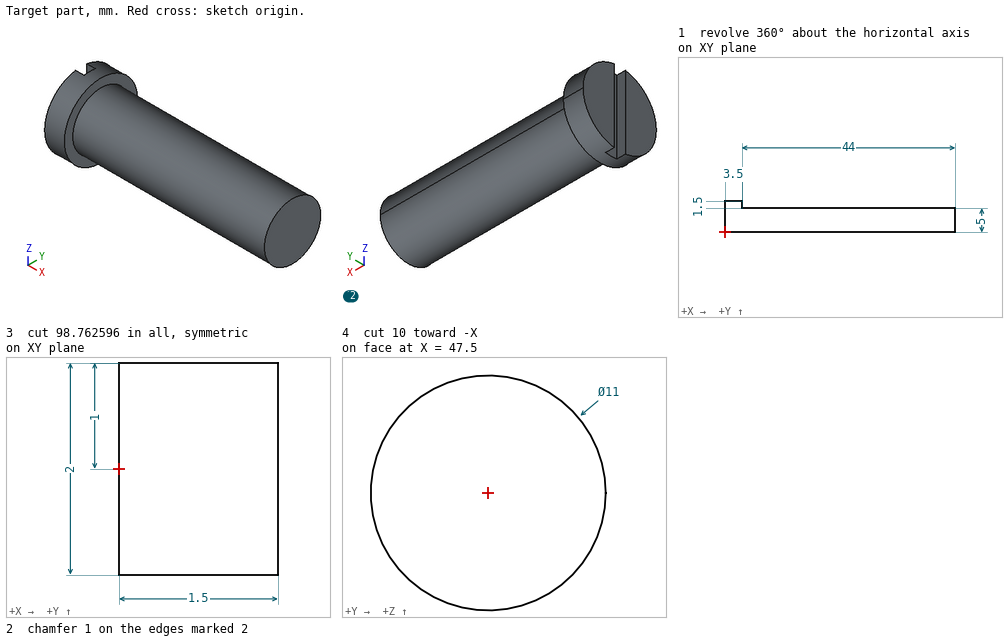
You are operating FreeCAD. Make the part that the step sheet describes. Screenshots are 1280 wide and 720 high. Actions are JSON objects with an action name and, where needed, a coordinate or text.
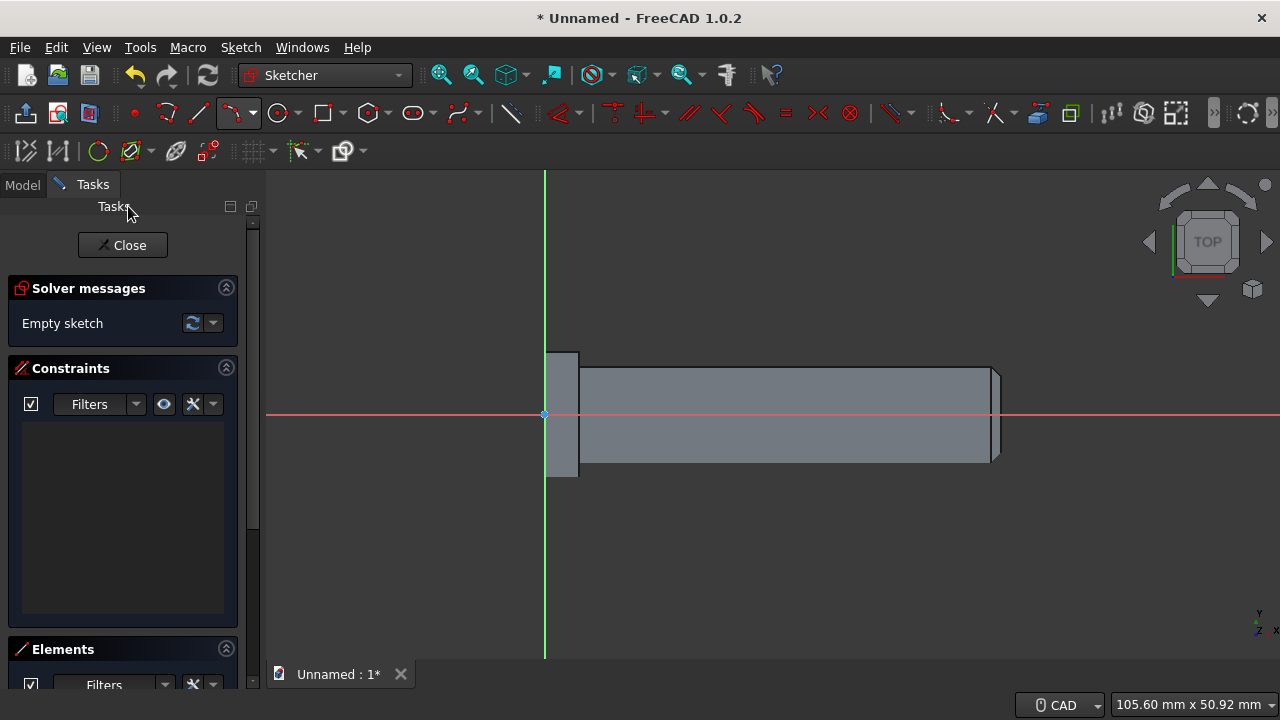
{"action": "scroll", "coordinate": [542, 415], "scroll_direction": "up", "scroll_amount": 14}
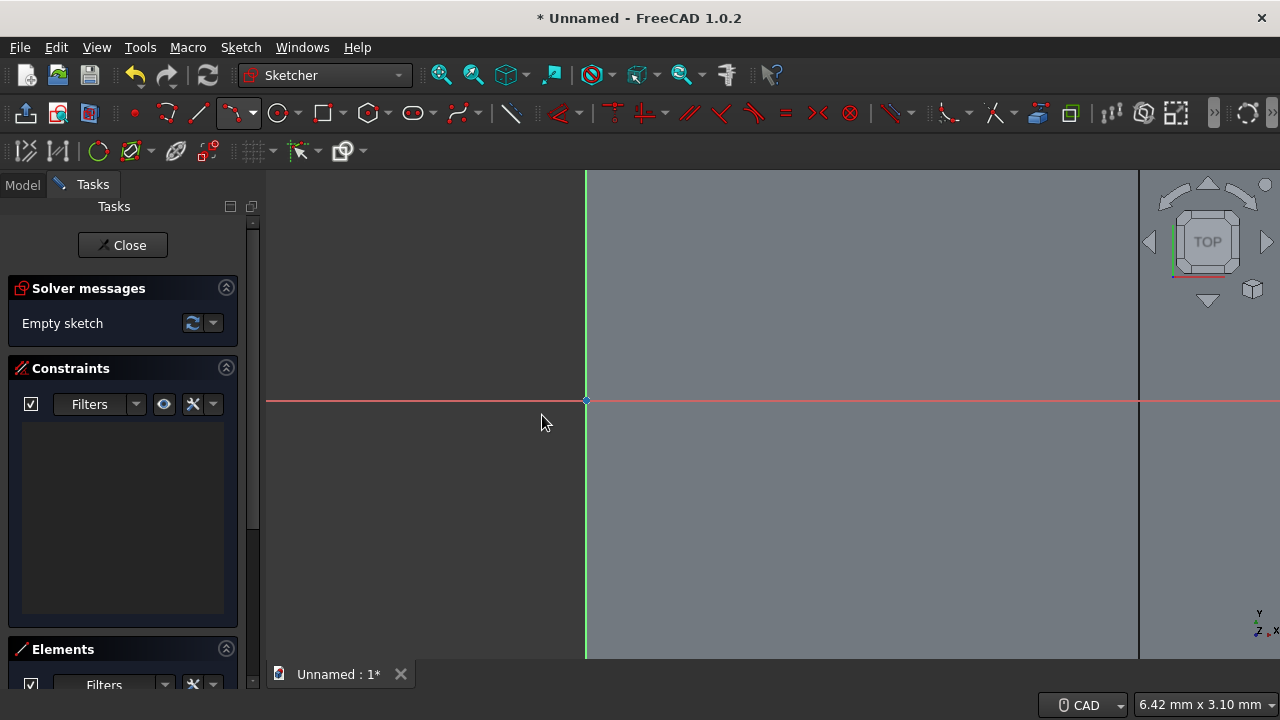
{"action": "key", "text": "g r"}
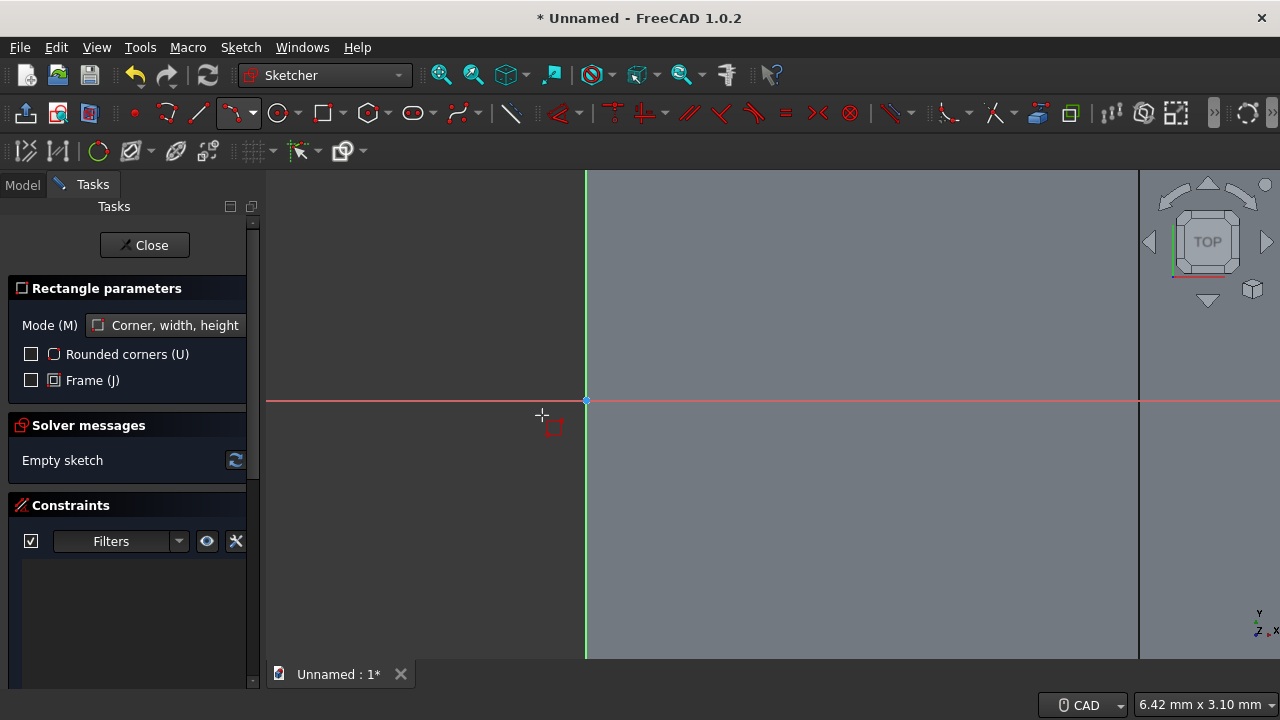
{"action": "left_click", "coordinate": [586, 243]}
{"action": "left_click", "coordinate": [823, 559]}
{"action": "key", "text": "Escape"}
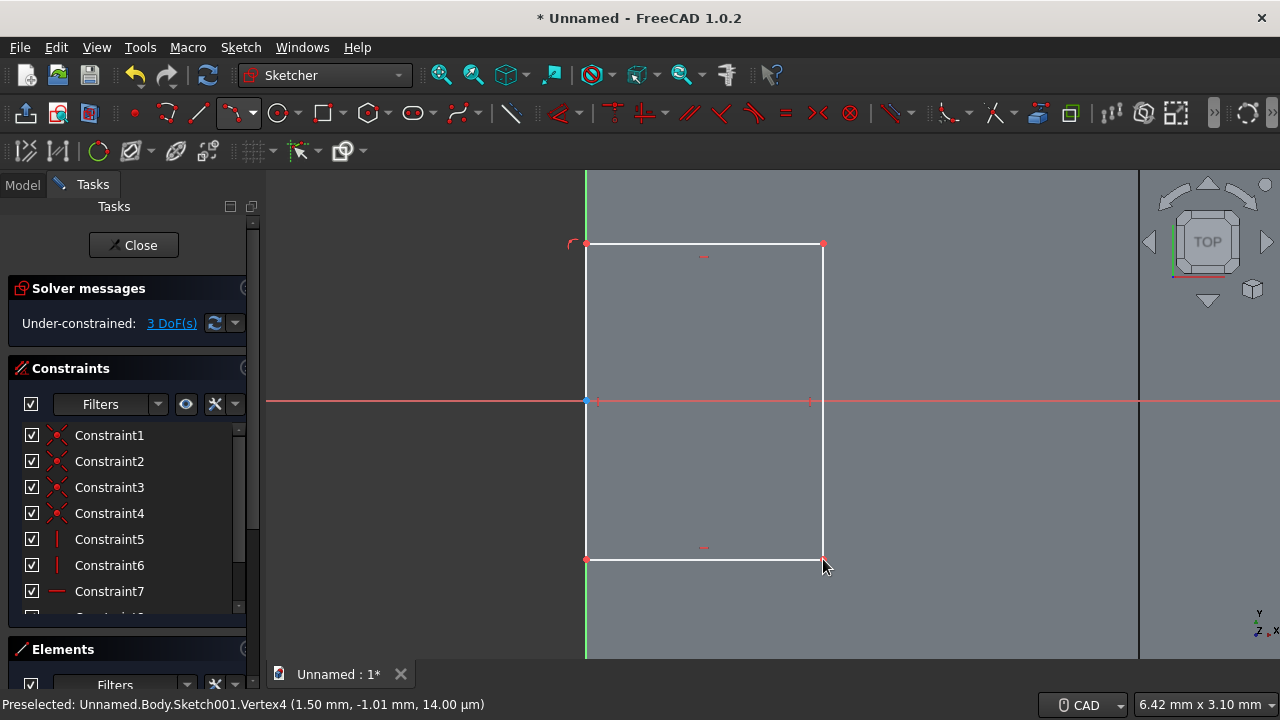
{"action": "key", "text": "d"}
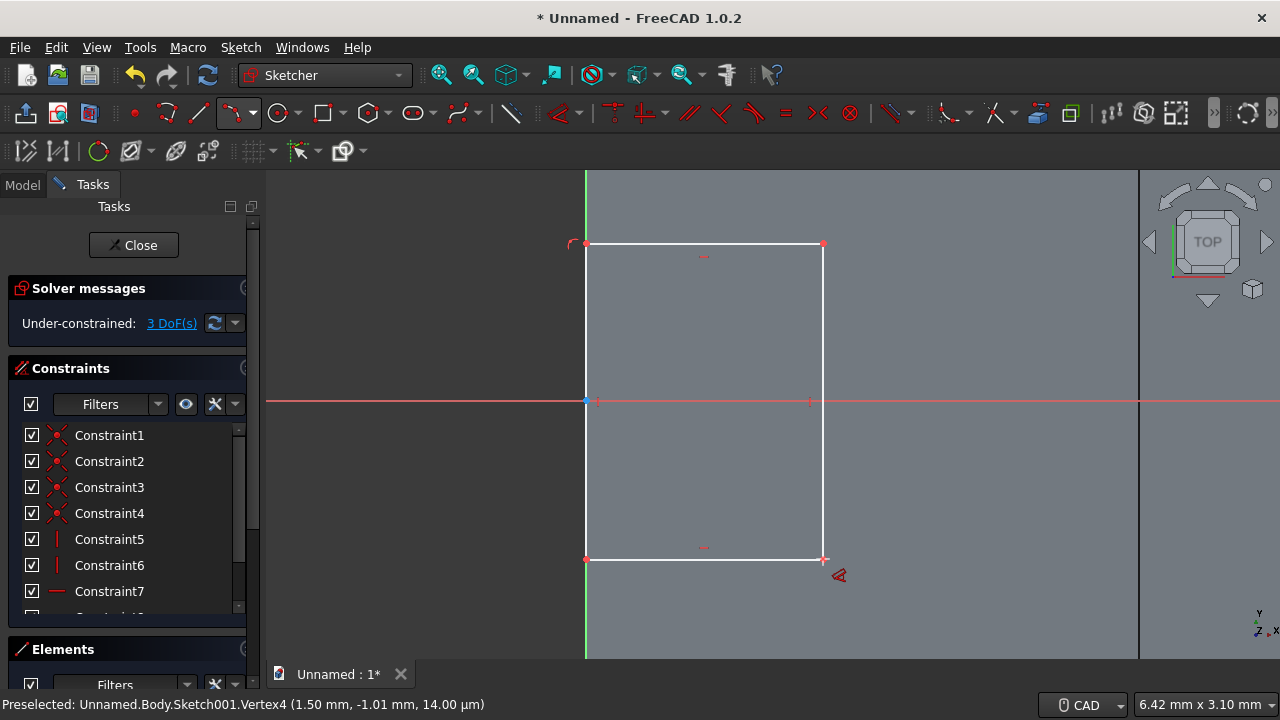
{"action": "left_click", "coordinate": [586, 339]}
{"action": "left_click", "coordinate": [552, 329]}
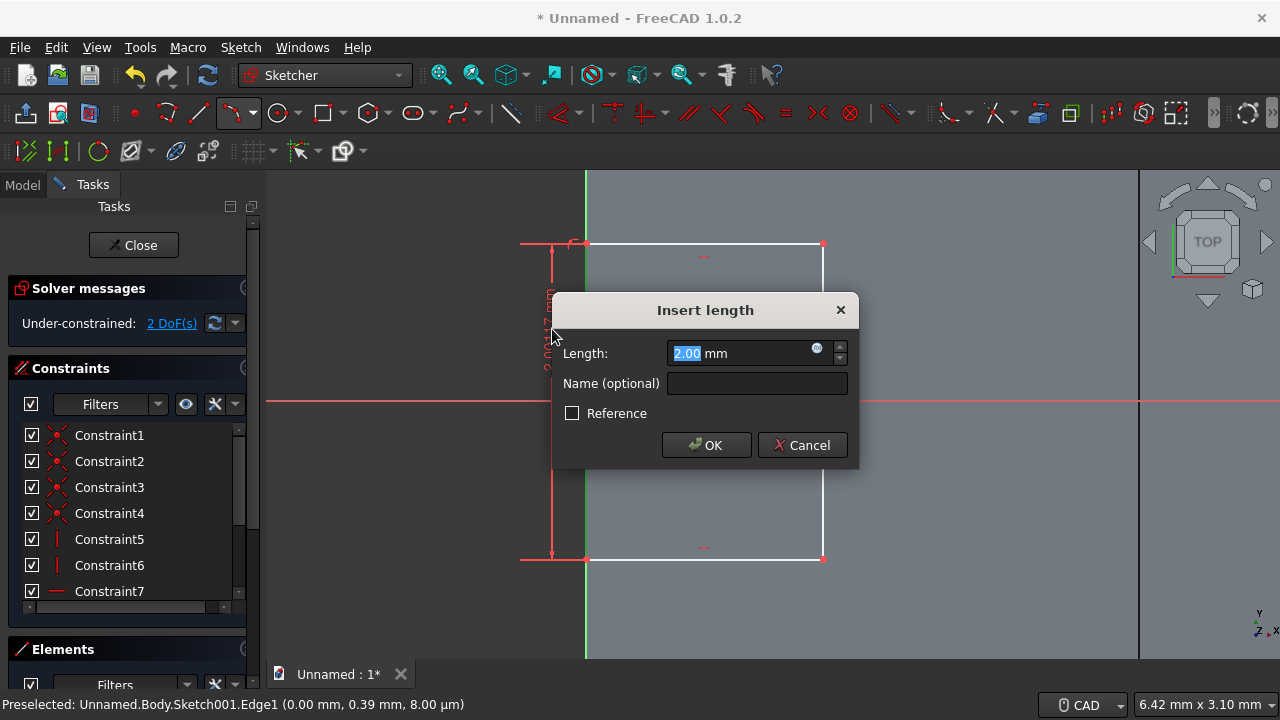
{"action": "type", "text": "2"}
{"action": "key", "text": "Return"}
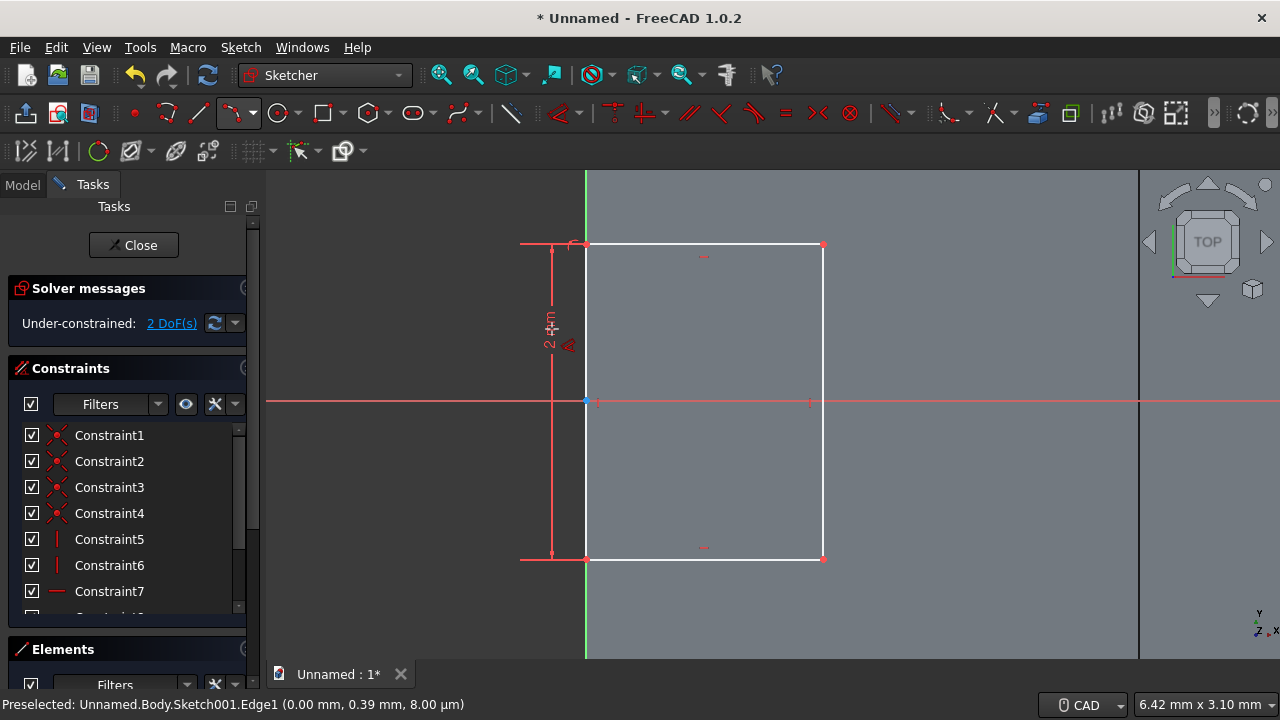
{"action": "left_click", "coordinate": [586, 244]}
{"action": "left_click", "coordinate": [552, 286]}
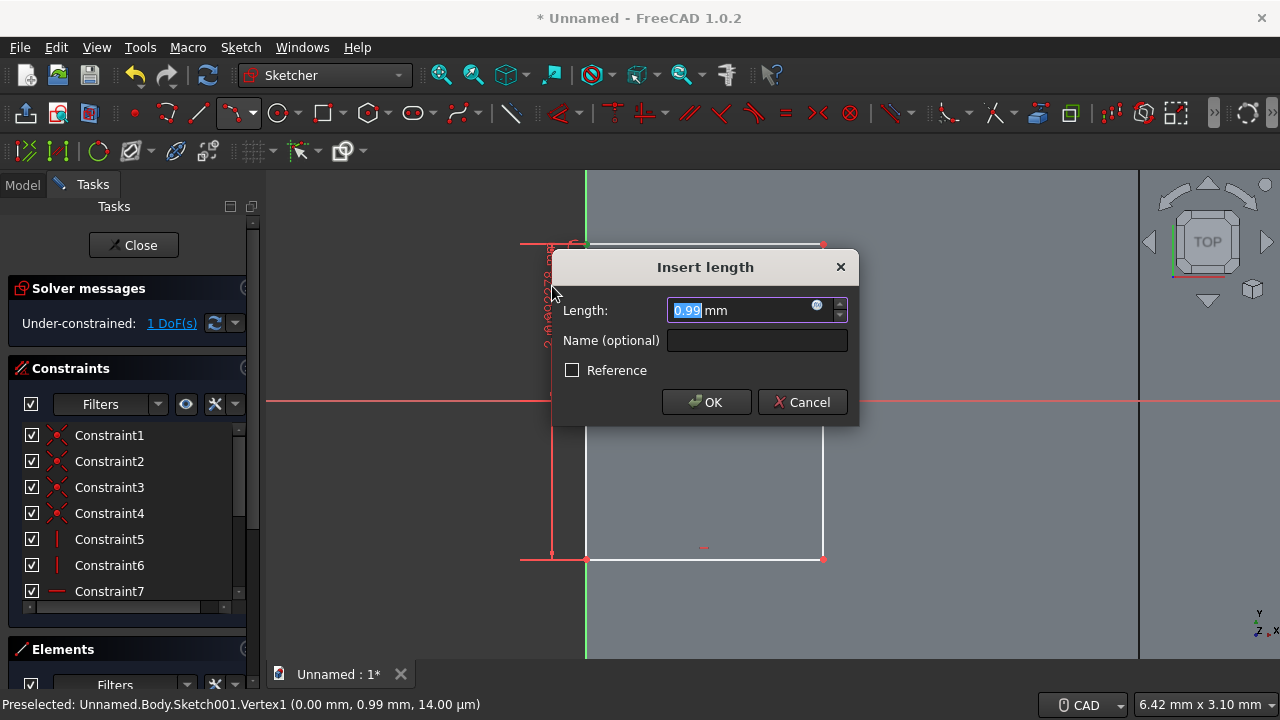
{"action": "type", "text": "1"}
{"action": "key", "text": "Return"}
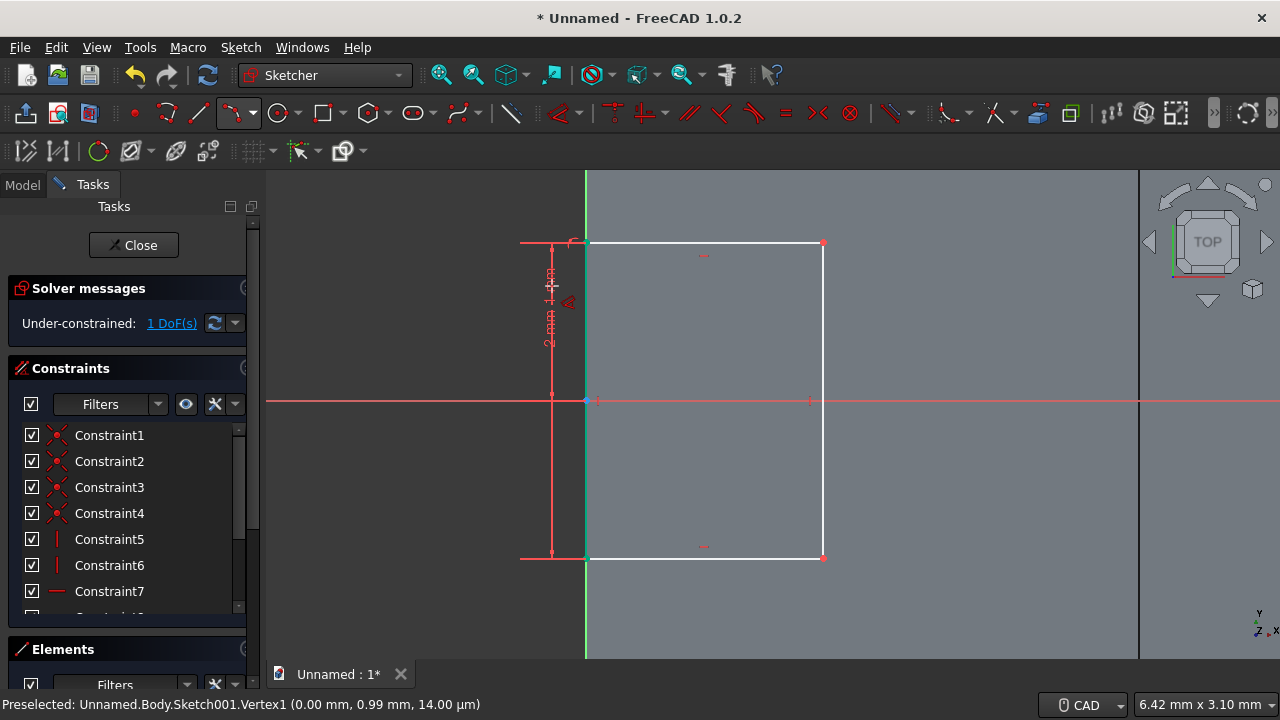
{"action": "left_click", "coordinate": [657, 559]}
{"action": "left_click", "coordinate": [705, 593]}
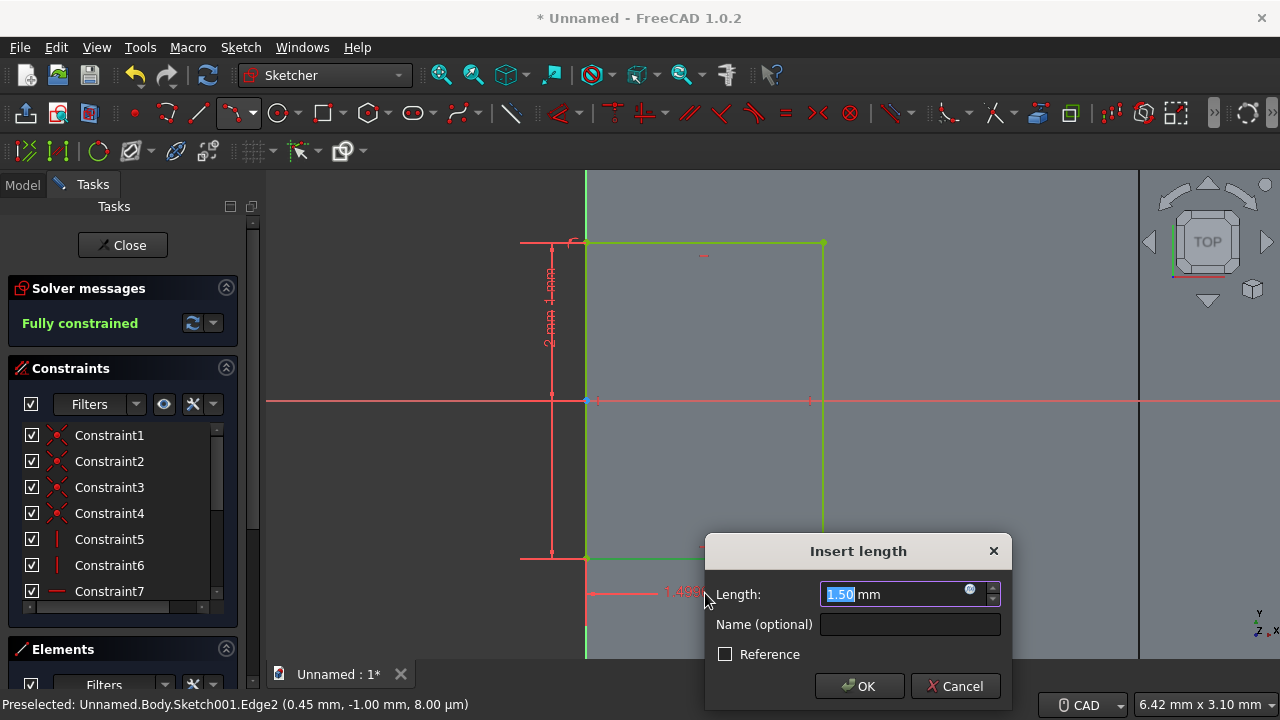
{"action": "type", "text": "1.5"}
{"action": "key", "text": "Return"}
{"action": "key", "text": "Escape"}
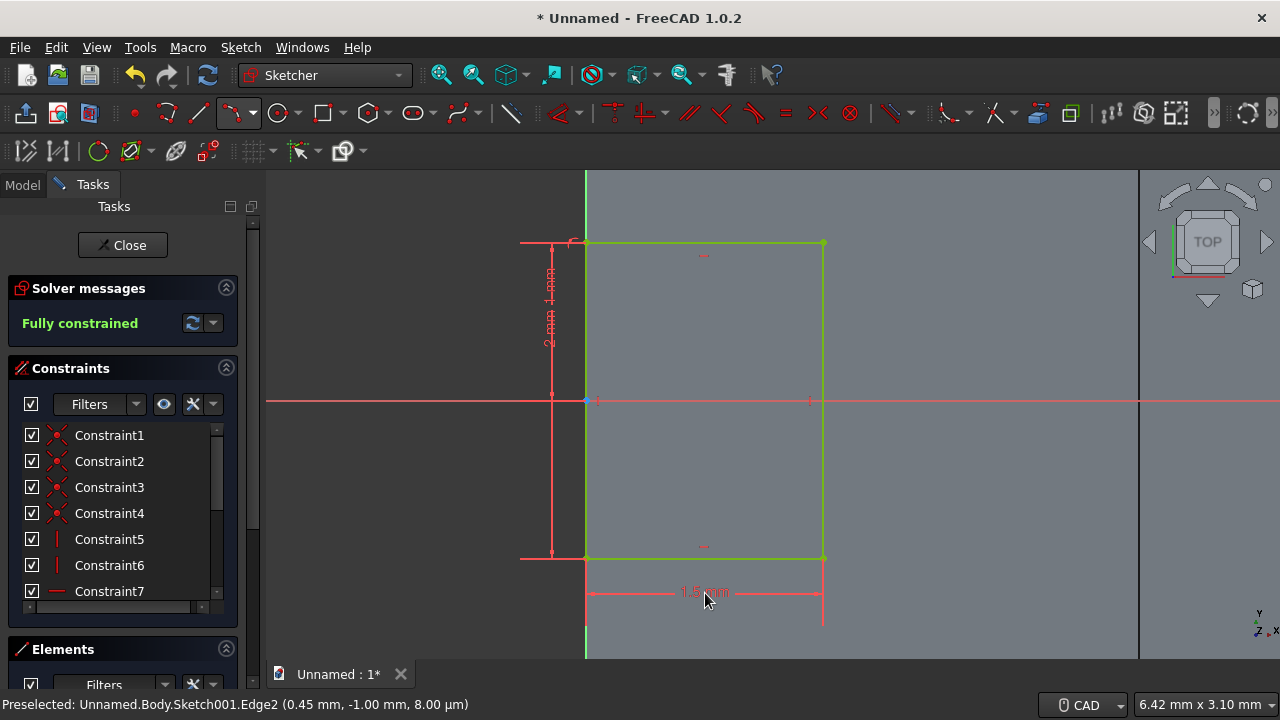
{"action": "left_click", "coordinate": [123, 245]}